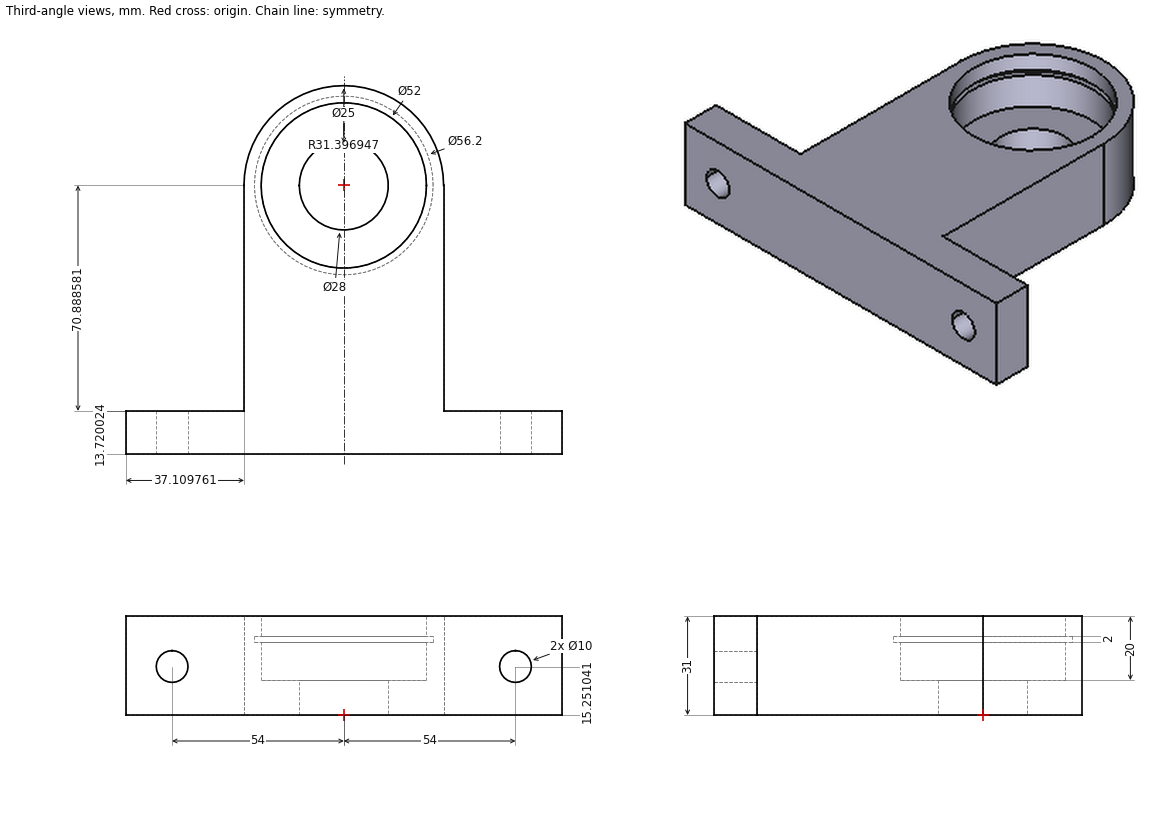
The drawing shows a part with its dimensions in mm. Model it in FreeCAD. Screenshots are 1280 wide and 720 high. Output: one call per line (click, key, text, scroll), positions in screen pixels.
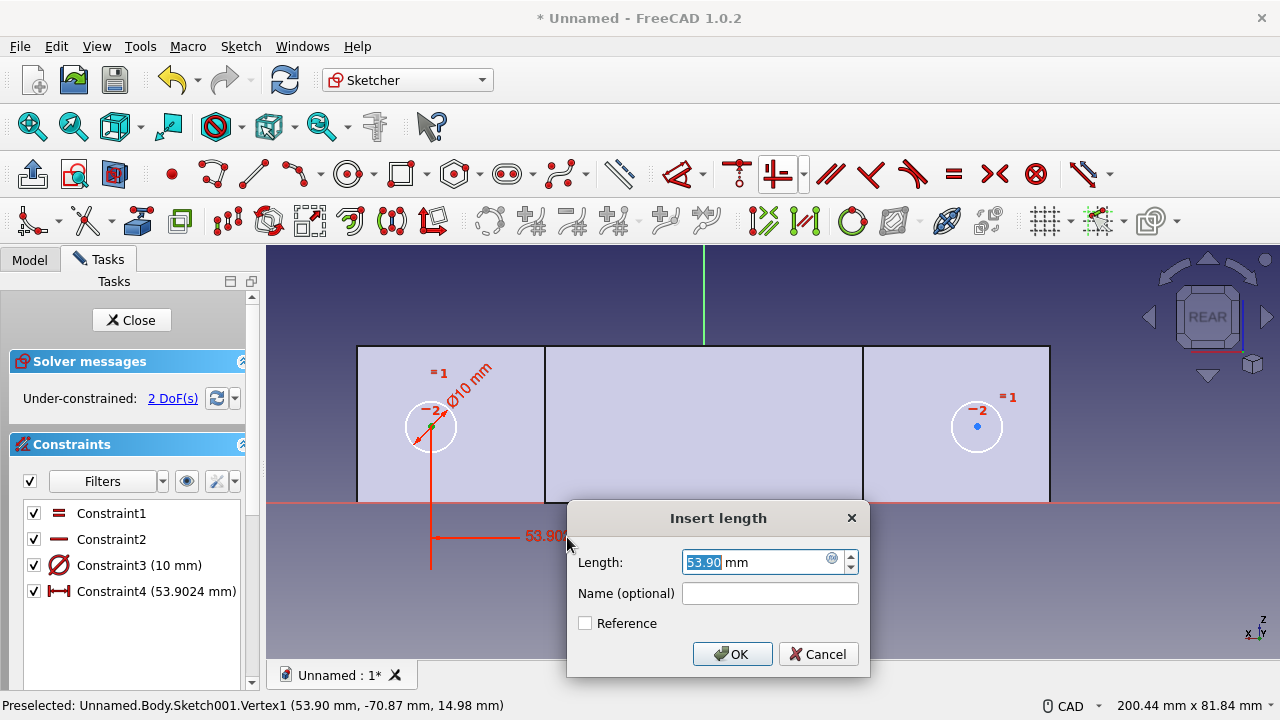
text(54)
key(Return)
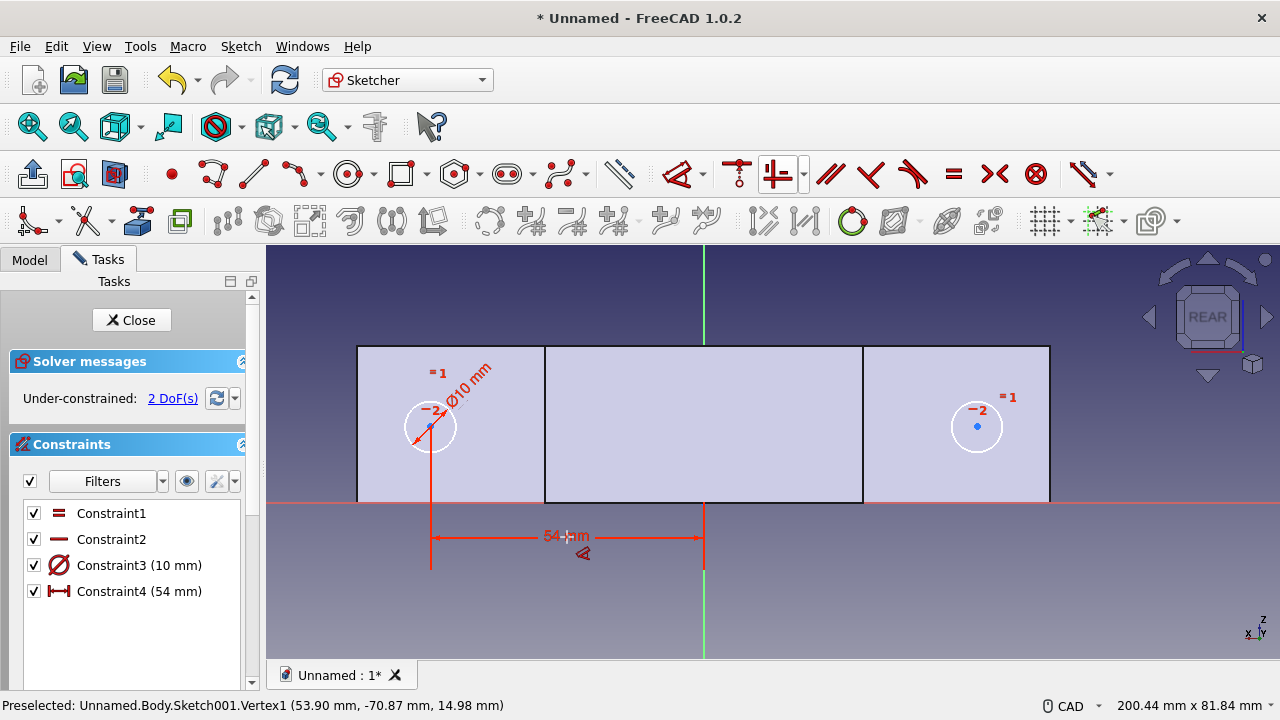
click(977, 427)
click(840, 537)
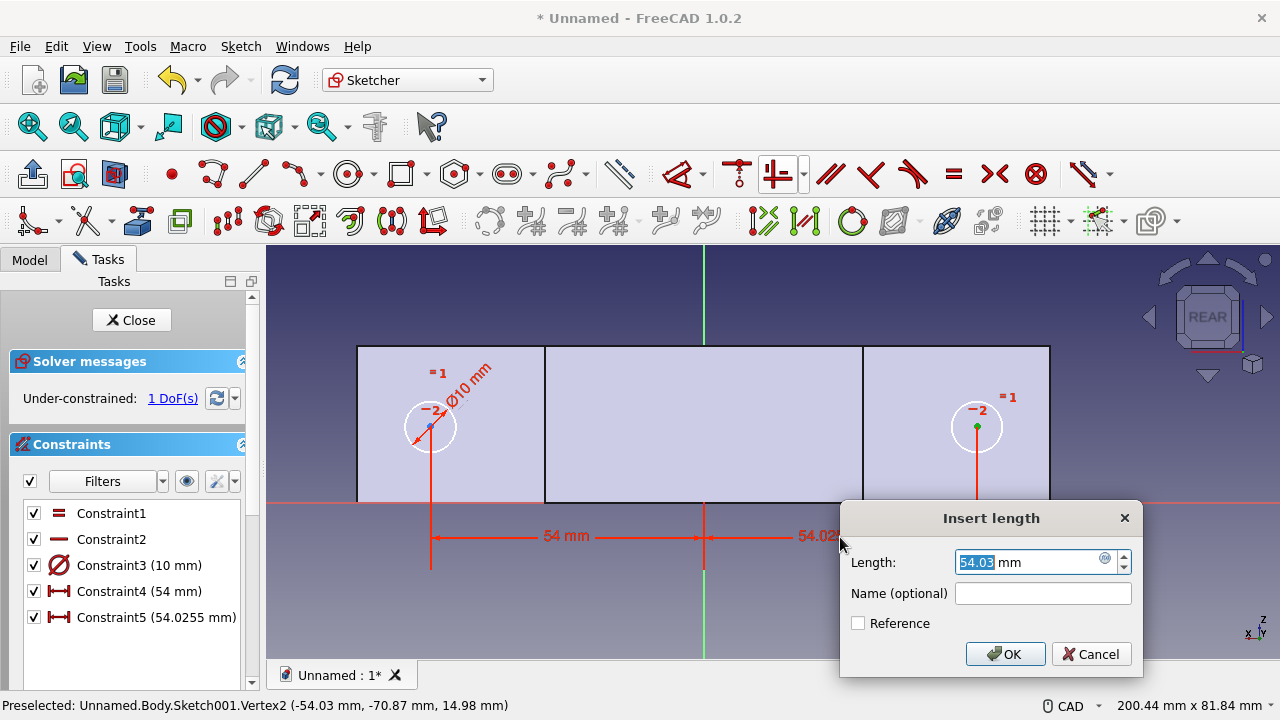
text(54)
key(Return)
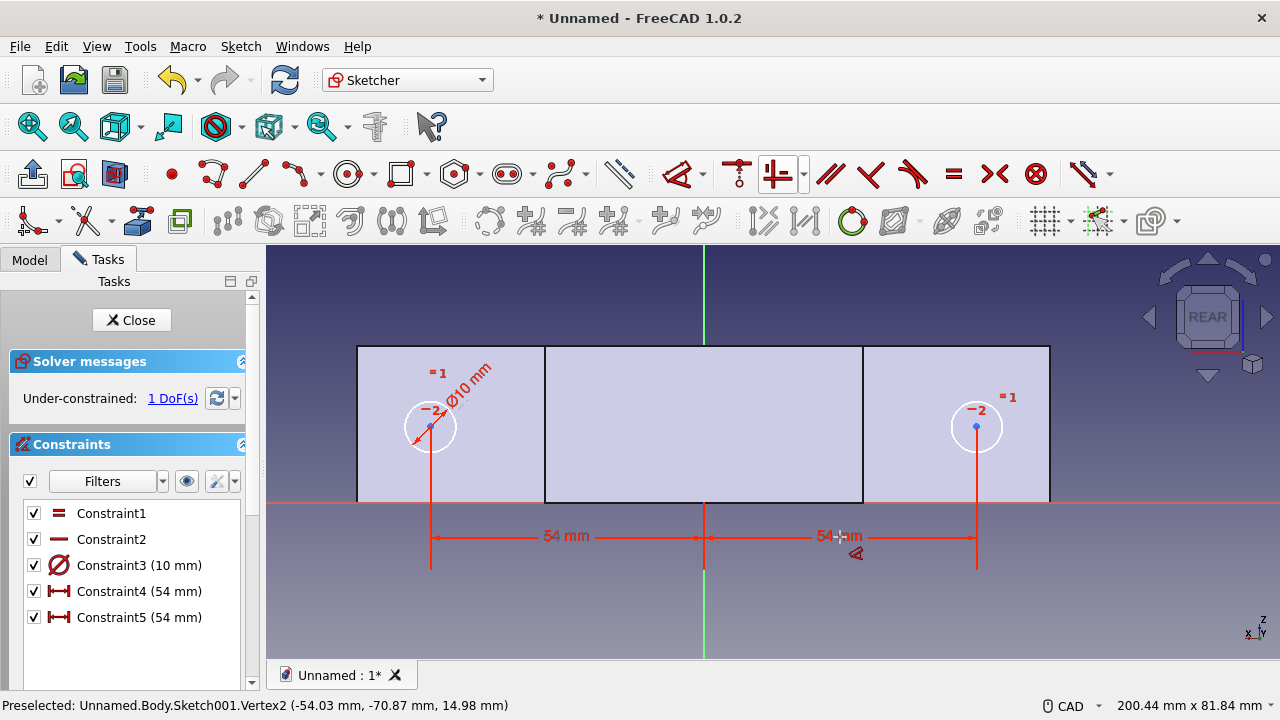
click(431, 427)
click(397, 465)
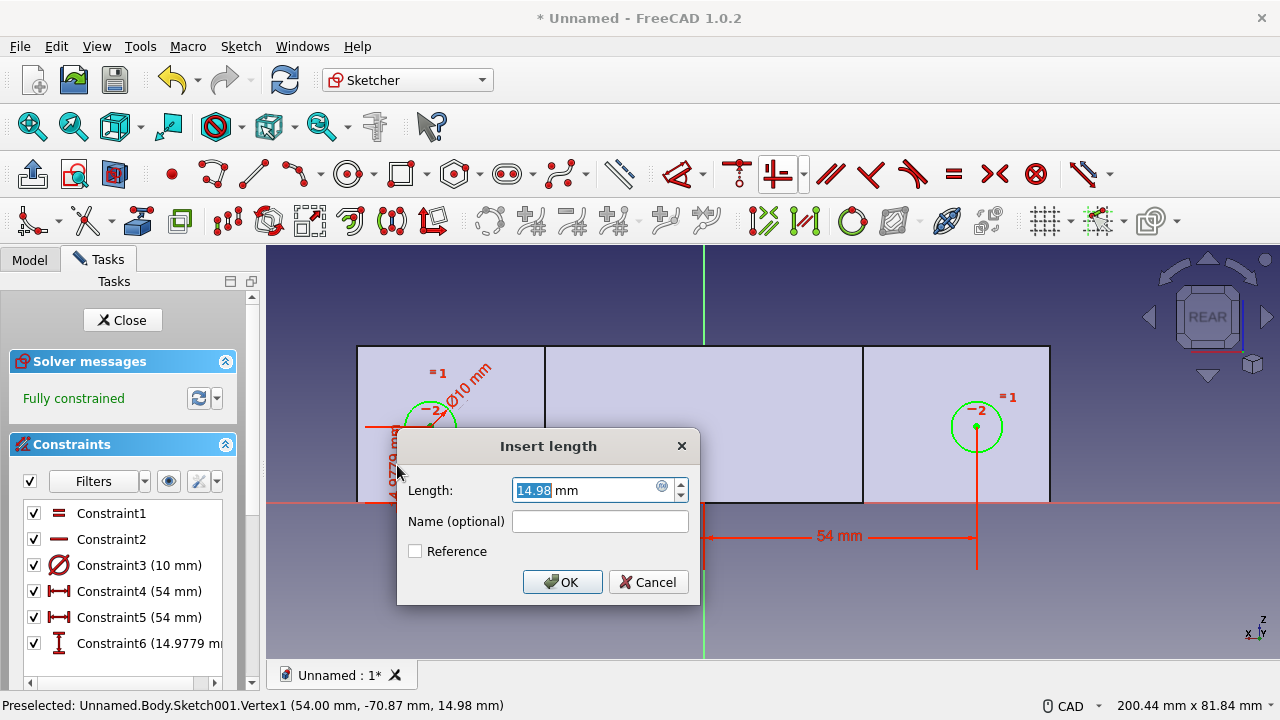
text(15.251041)
key(Return)
key(Escape)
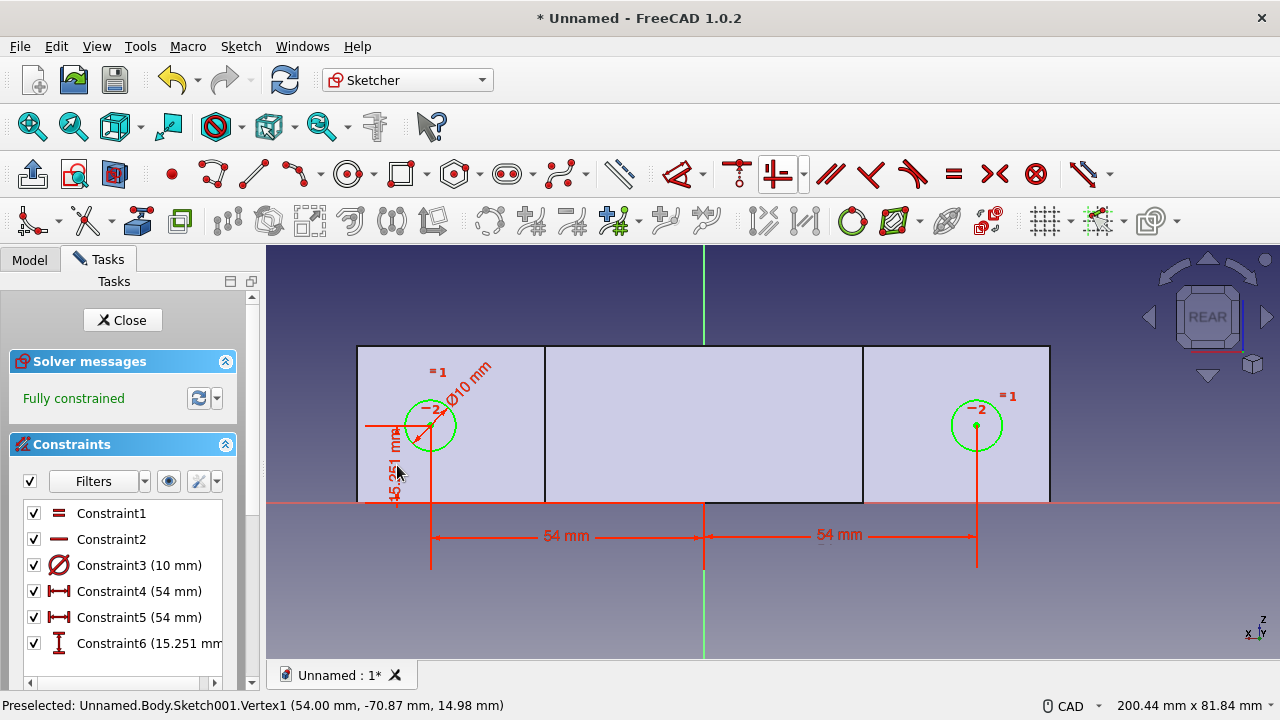
click(123, 320)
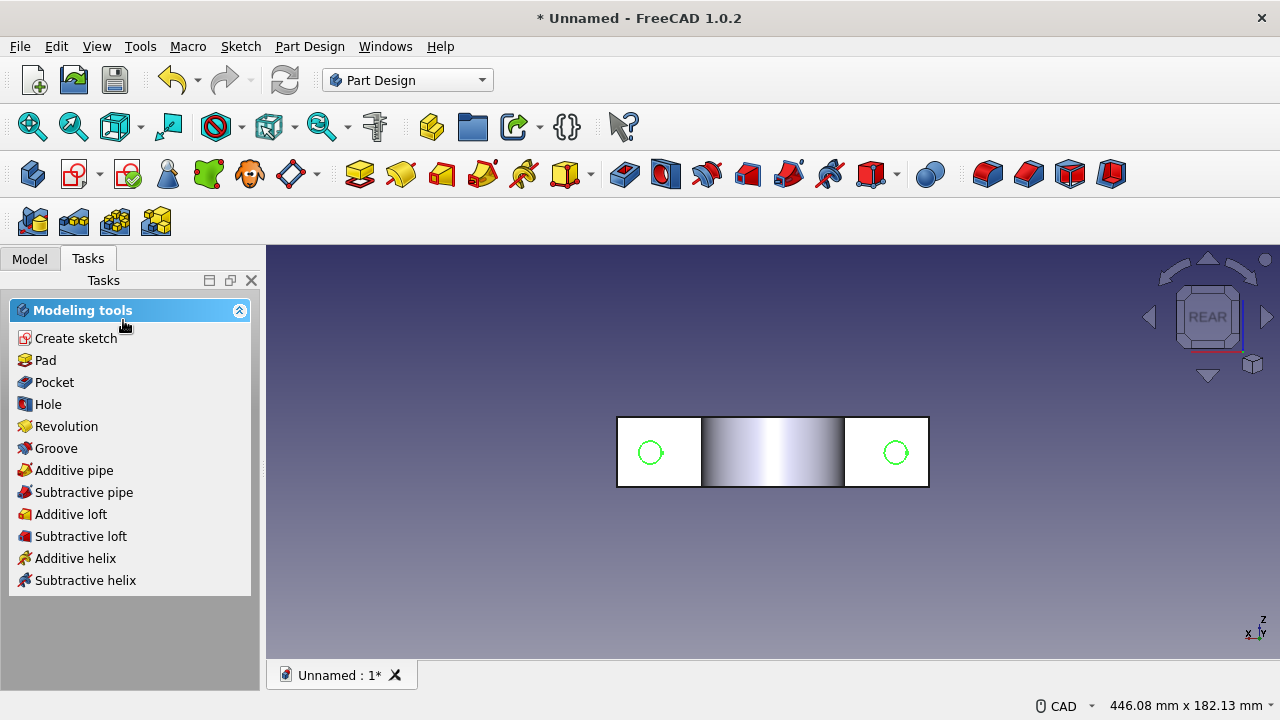
click(625, 174)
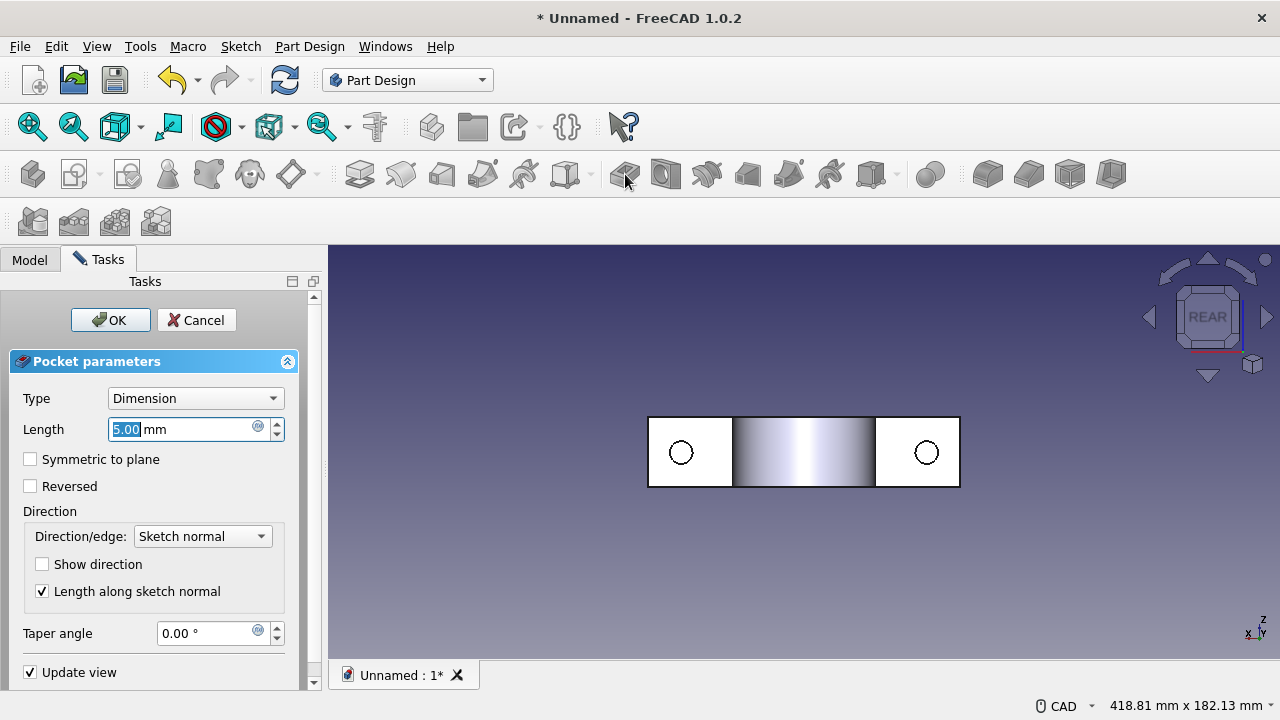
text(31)
key(Tab)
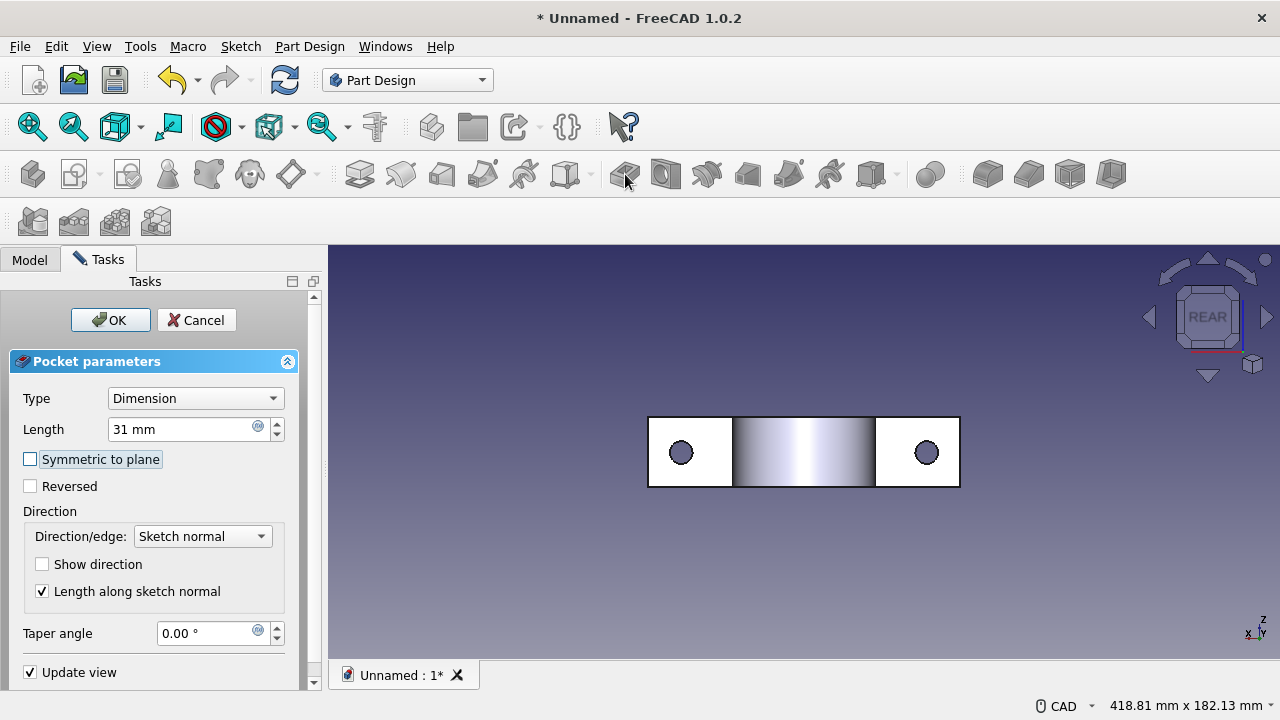
click(111, 320)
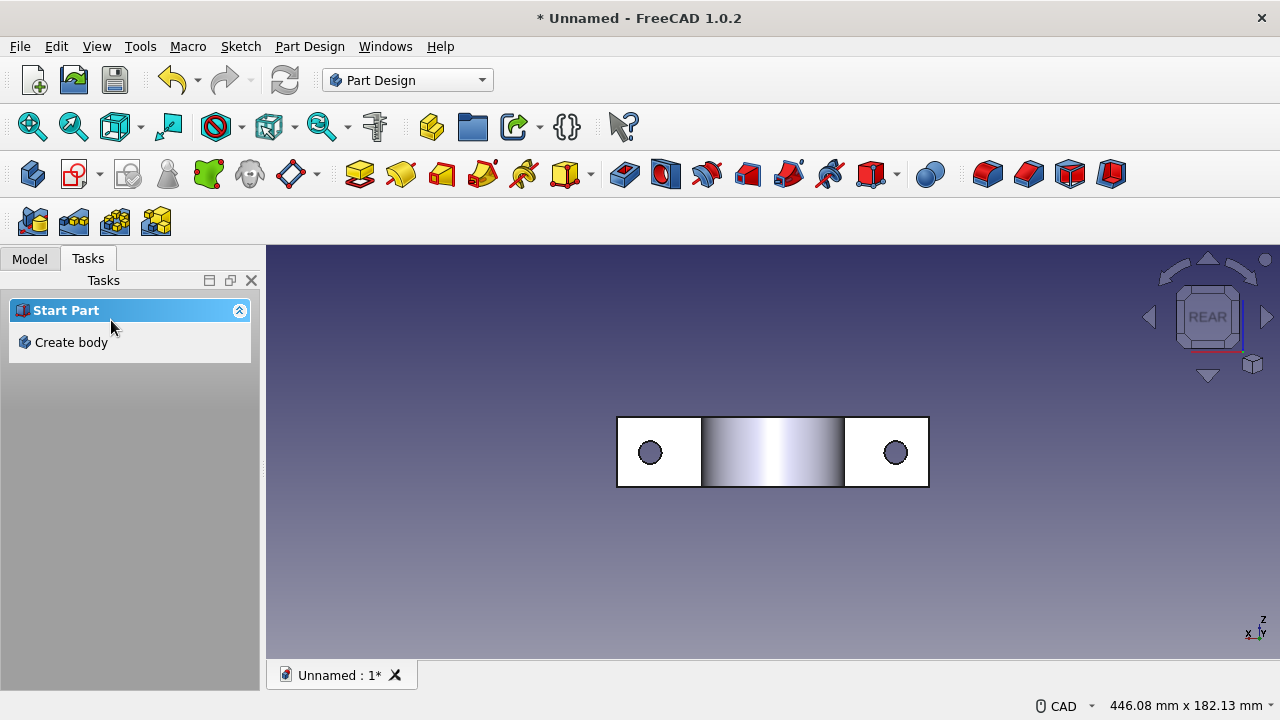
click(33, 128)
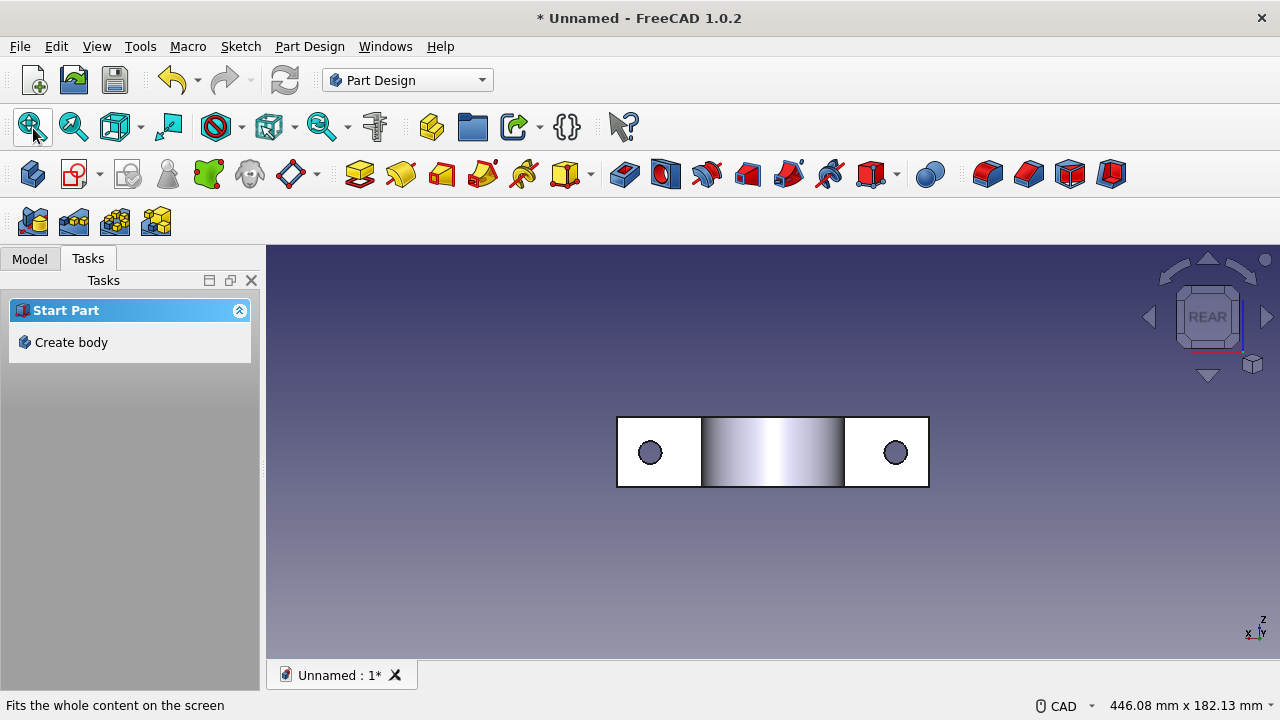
click(74, 174)